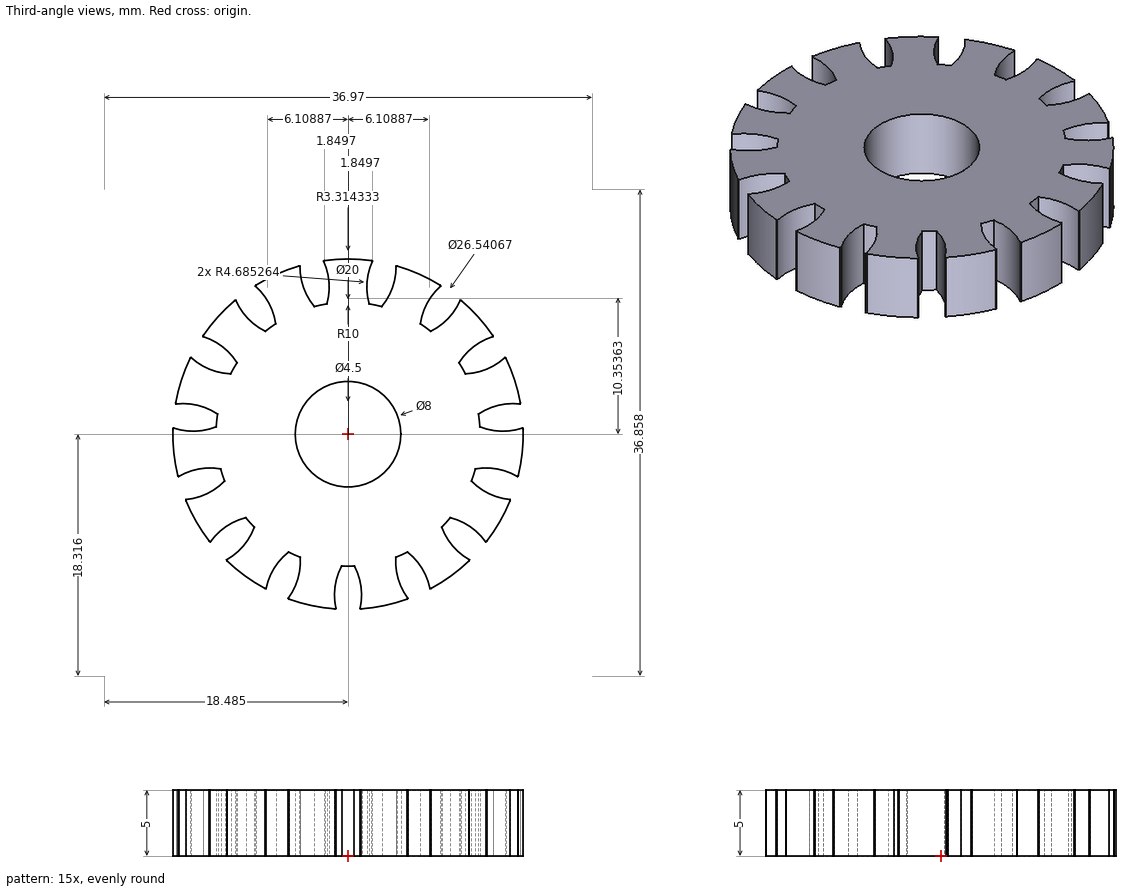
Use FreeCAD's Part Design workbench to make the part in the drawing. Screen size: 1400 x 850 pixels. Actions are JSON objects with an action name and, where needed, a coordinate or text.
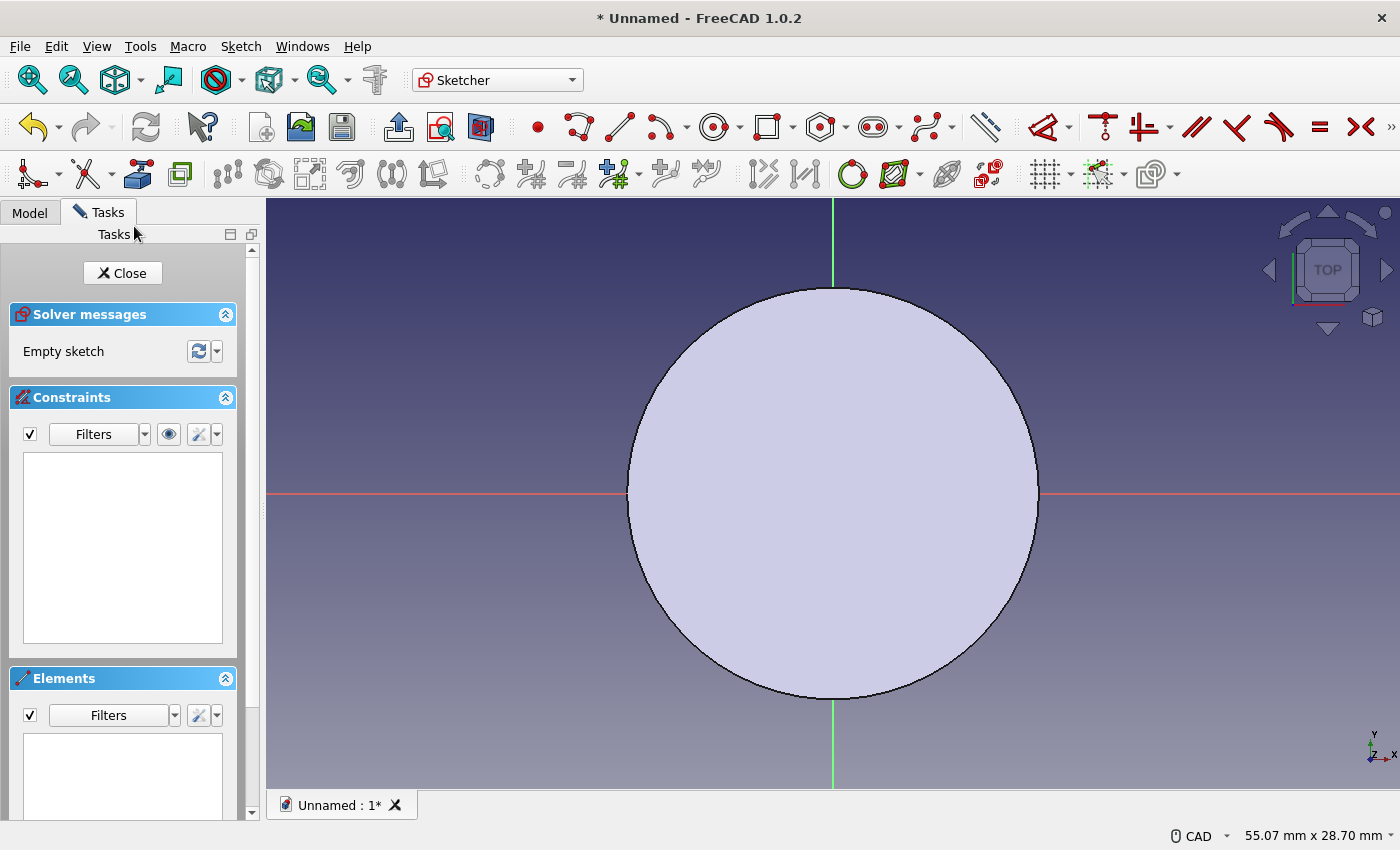
{"action": "left_click", "coordinate": [481, 128]}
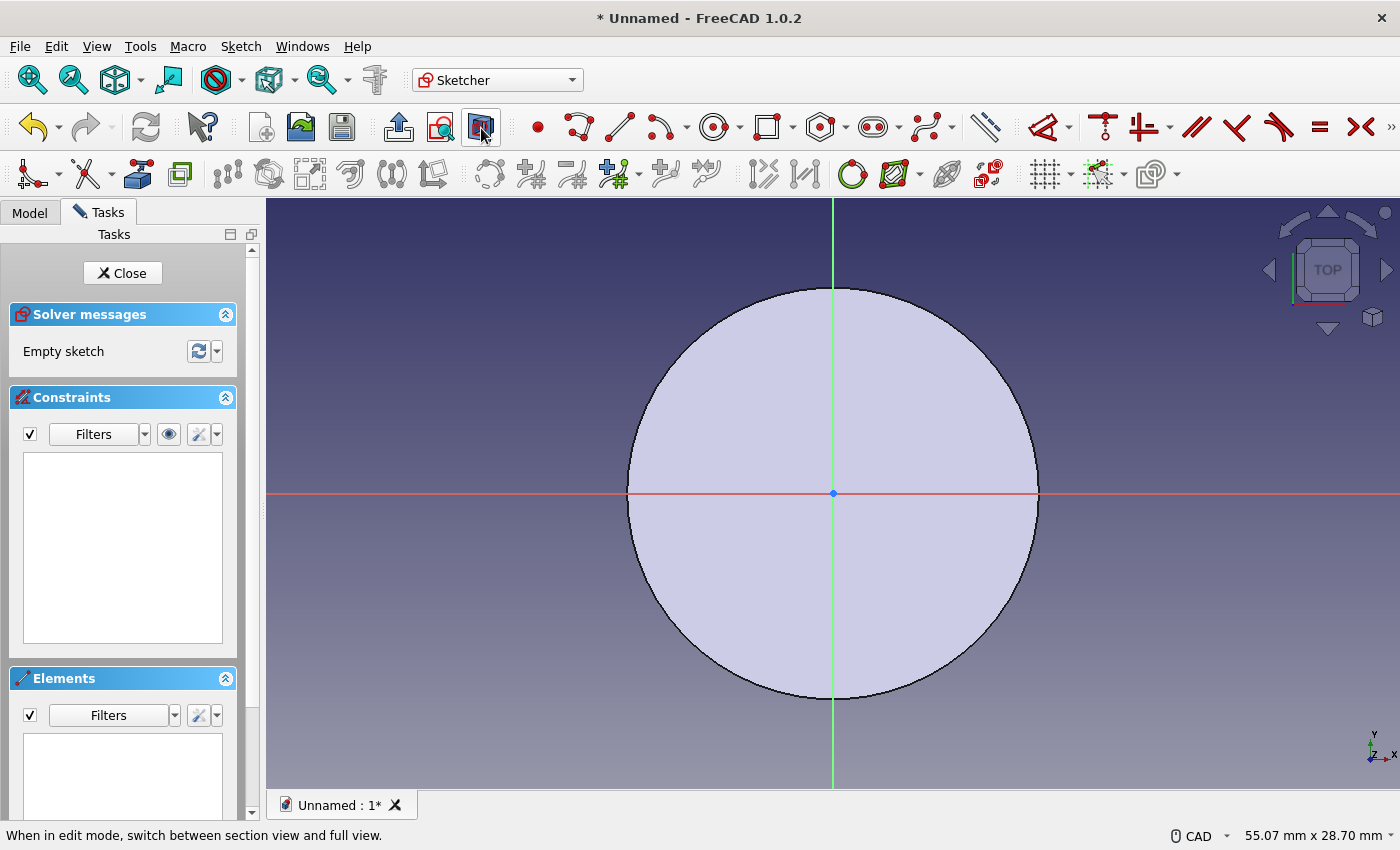
{"action": "scroll", "coordinate": [855, 494], "scroll_direction": "up", "scroll_amount": 7}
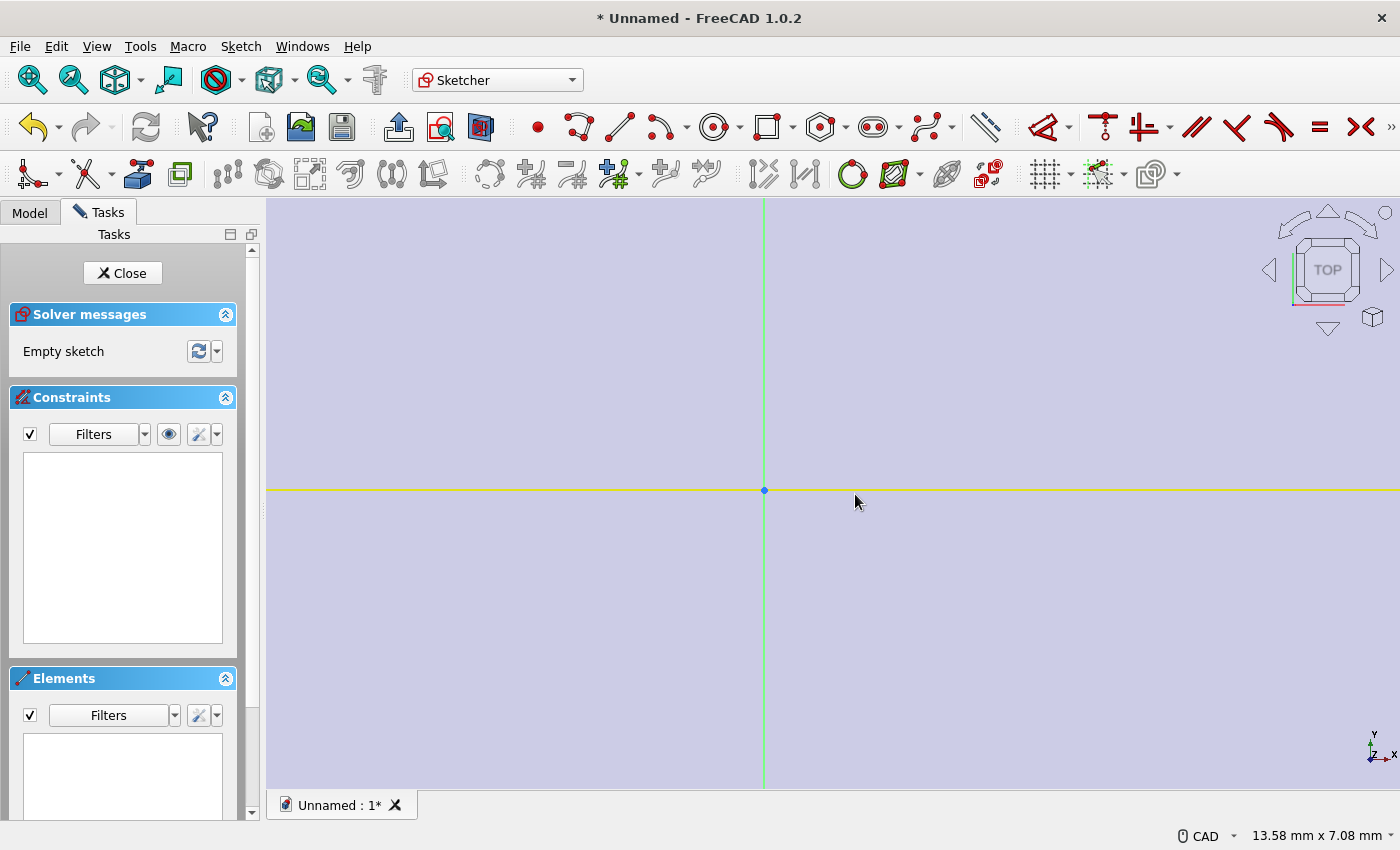
{"action": "key", "text": "g c"}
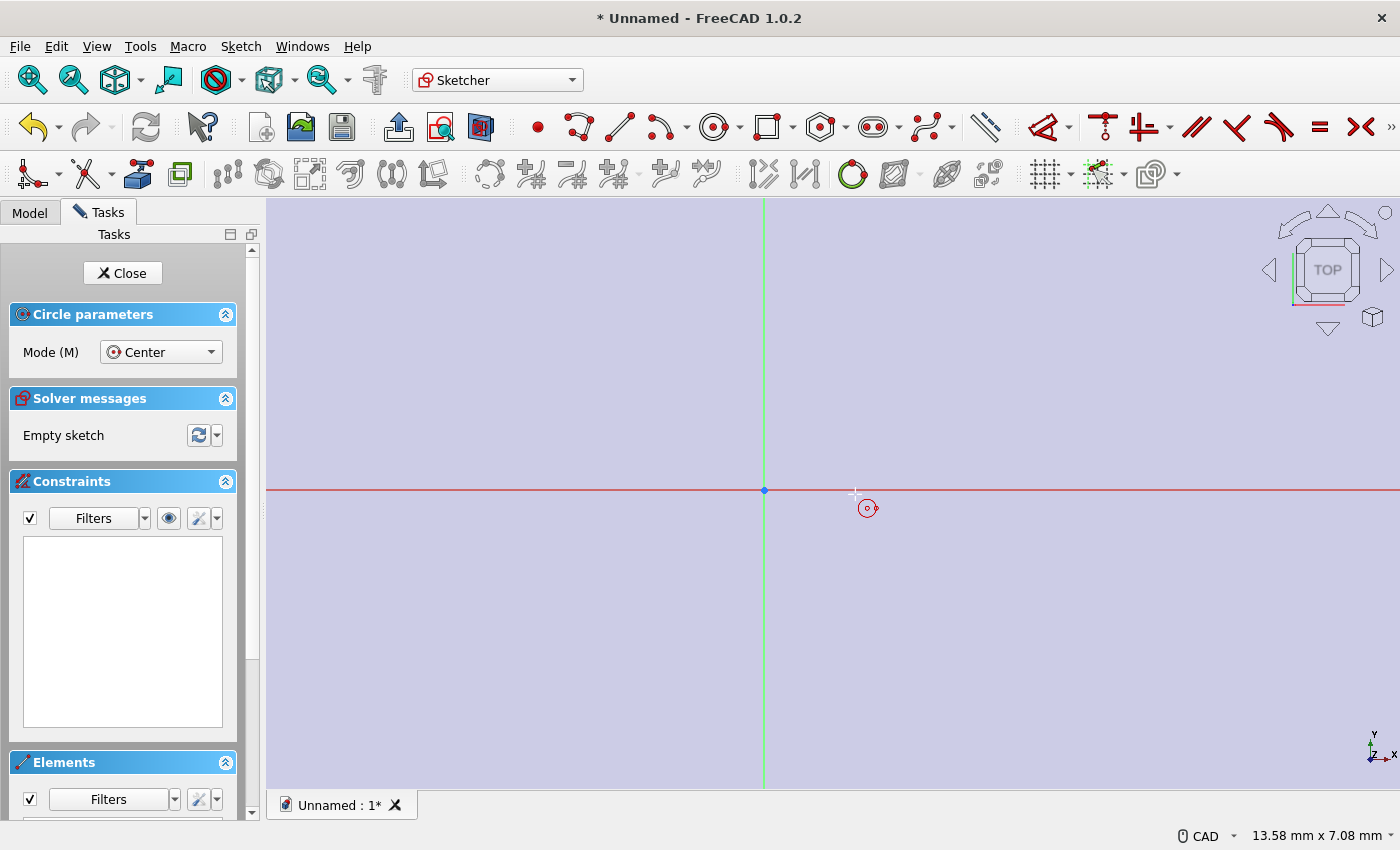
{"action": "left_click", "coordinate": [764, 490]}
{"action": "mouse_move", "coordinate": [897, 358]}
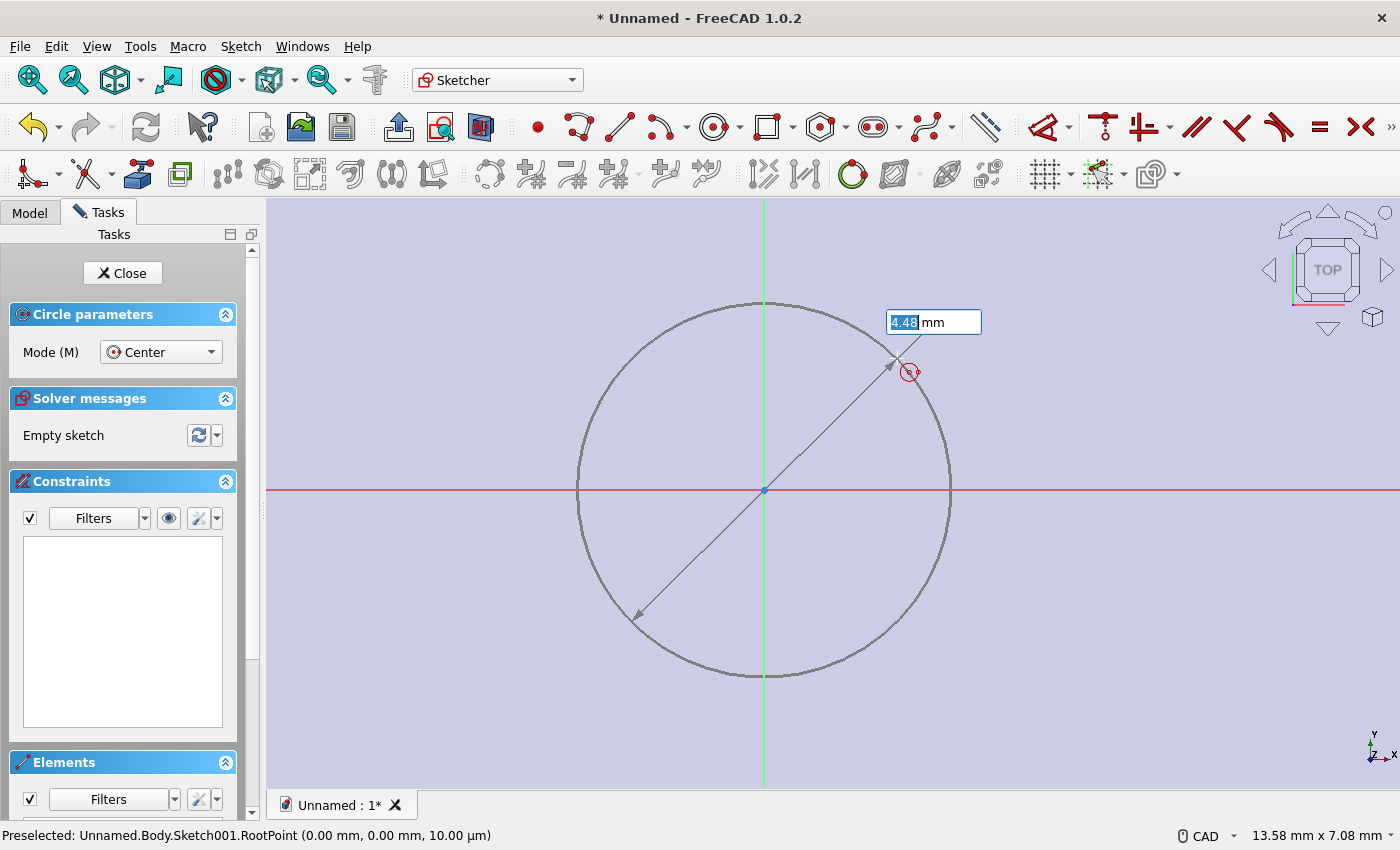
{"action": "type", "text": "4.5"}
{"action": "key", "text": "Return"}
{"action": "key", "text": "Escape"}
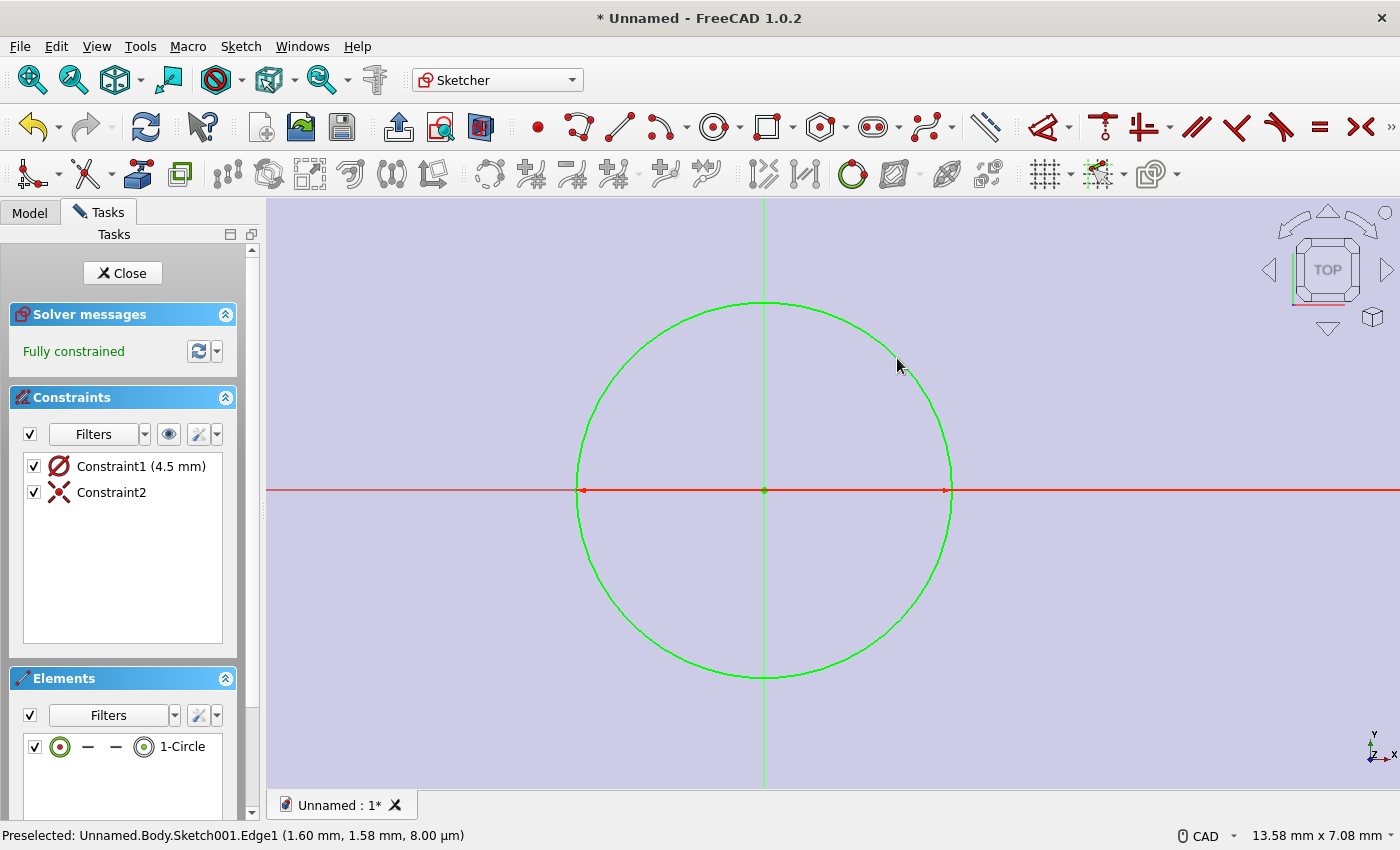
{"action": "left_click", "coordinate": [123, 273]}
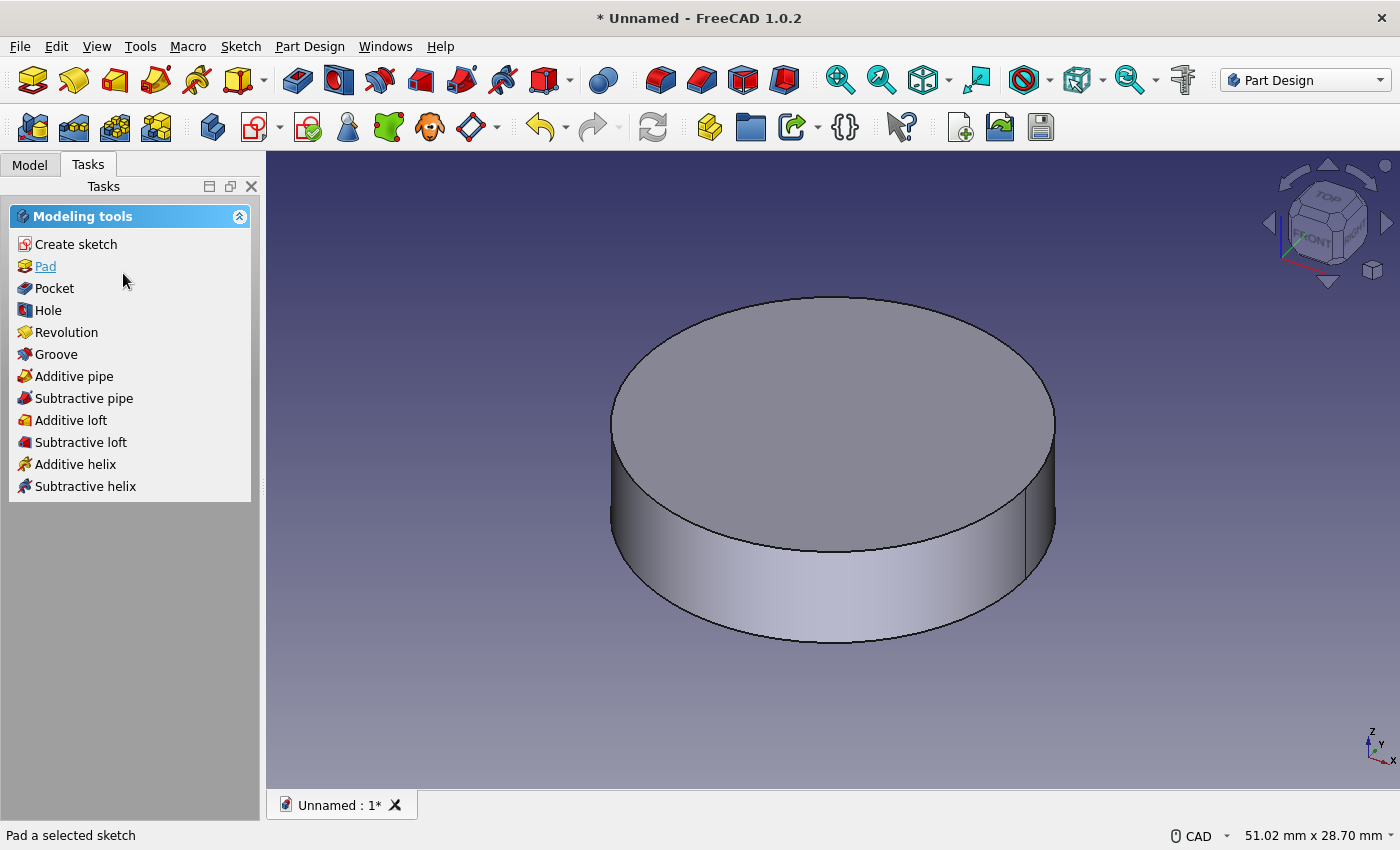
{"action": "left_click", "coordinate": [298, 80]}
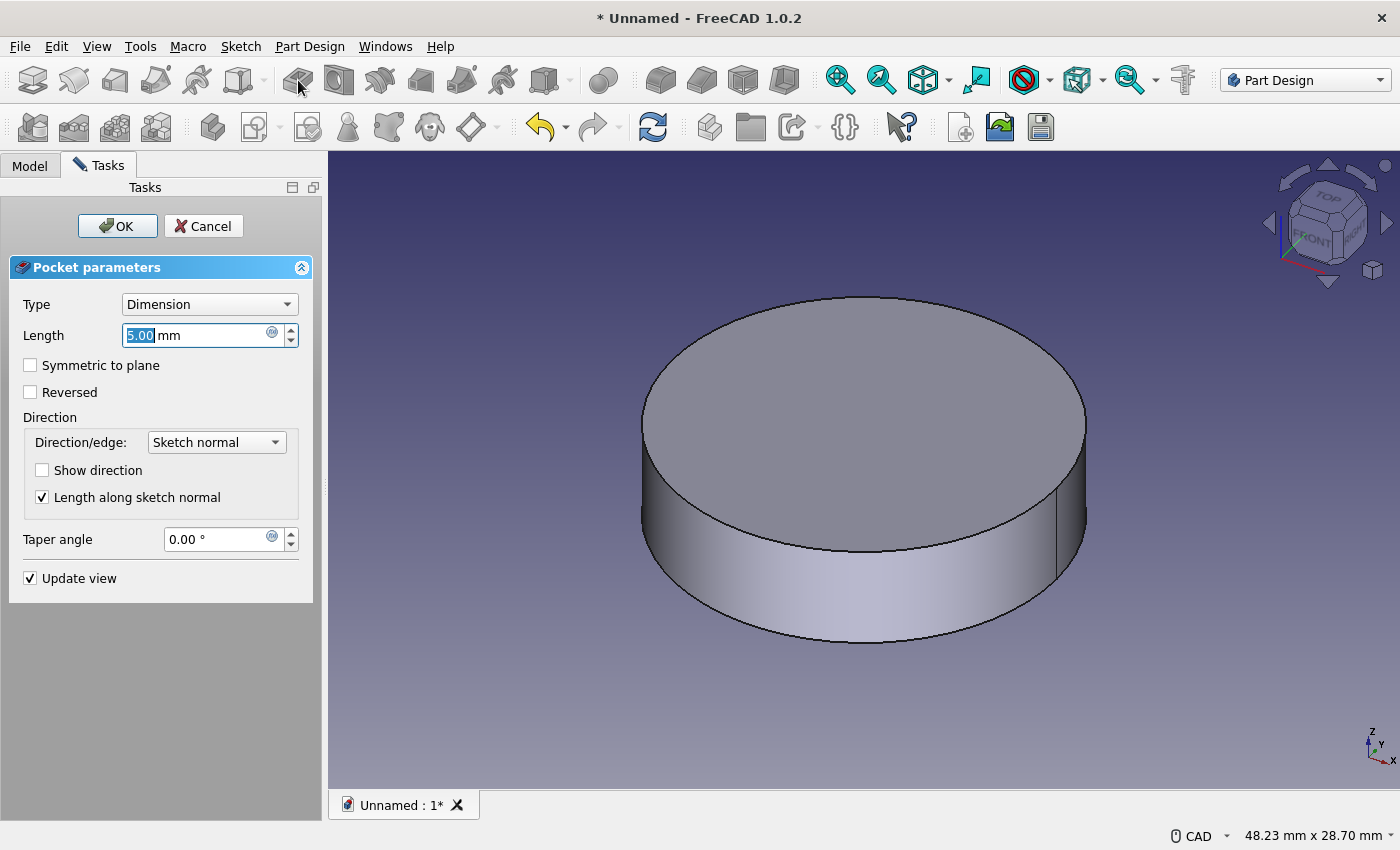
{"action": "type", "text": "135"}
{"action": "key", "text": "Tab"}